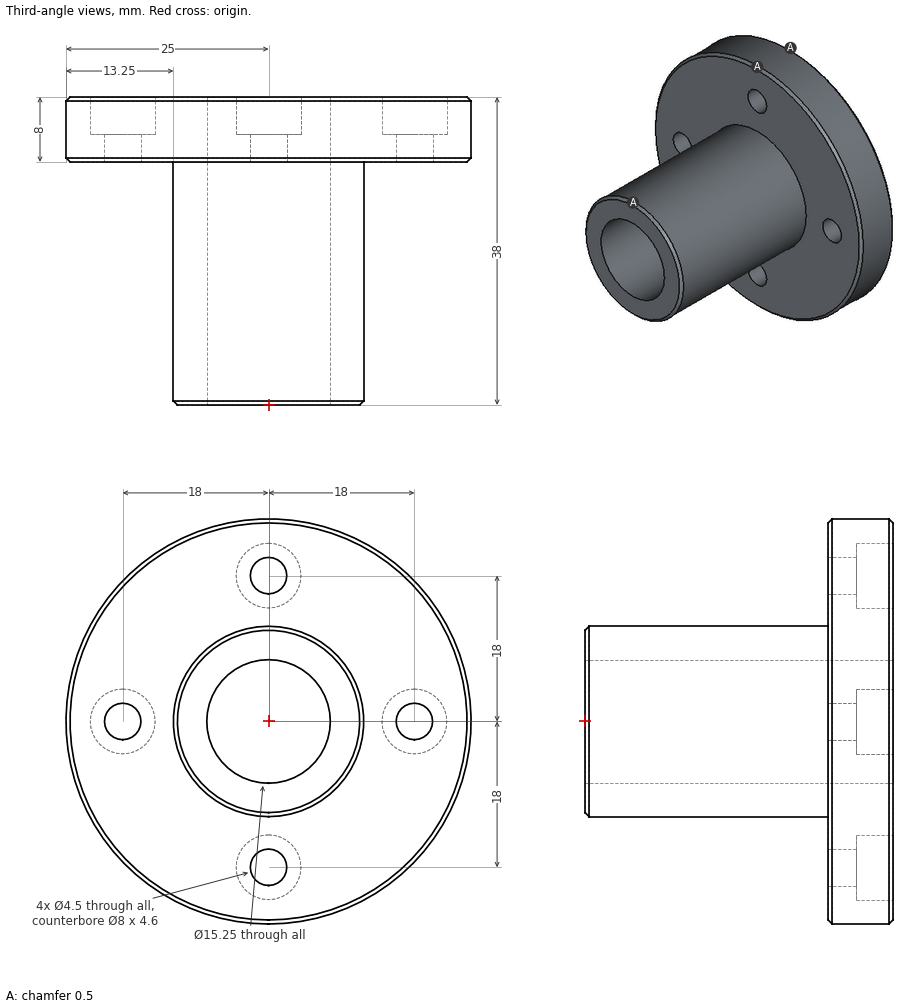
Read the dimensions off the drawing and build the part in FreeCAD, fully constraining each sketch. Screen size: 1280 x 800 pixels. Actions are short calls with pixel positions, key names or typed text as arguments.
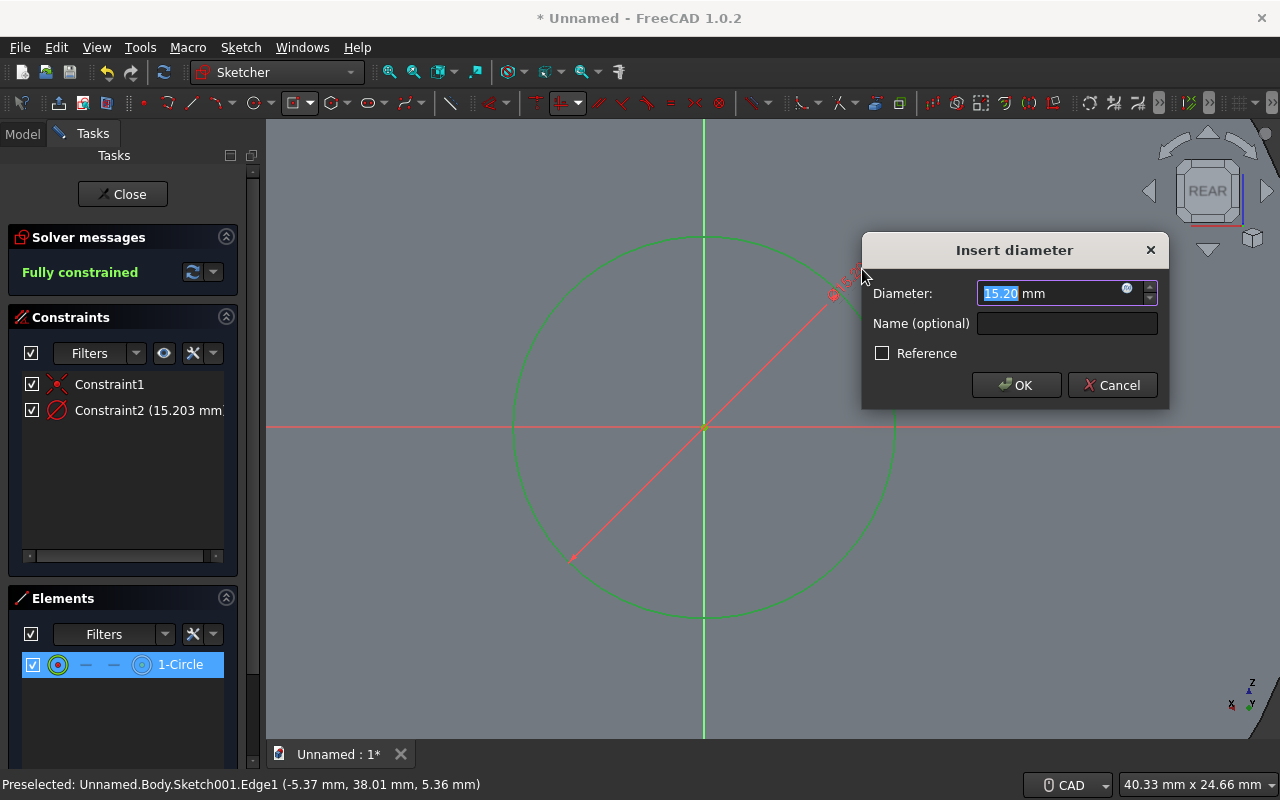
text(15.25)
key(Return)
key(Escape)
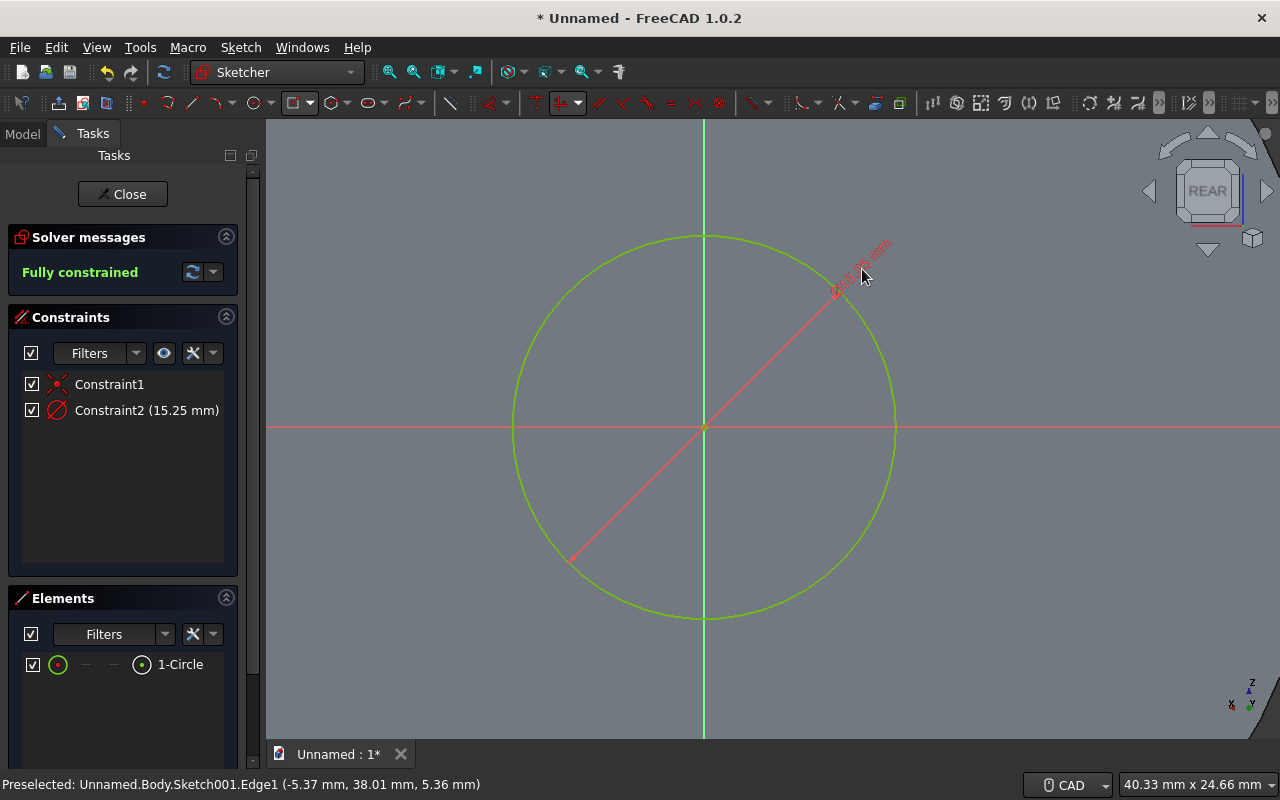
click(123, 194)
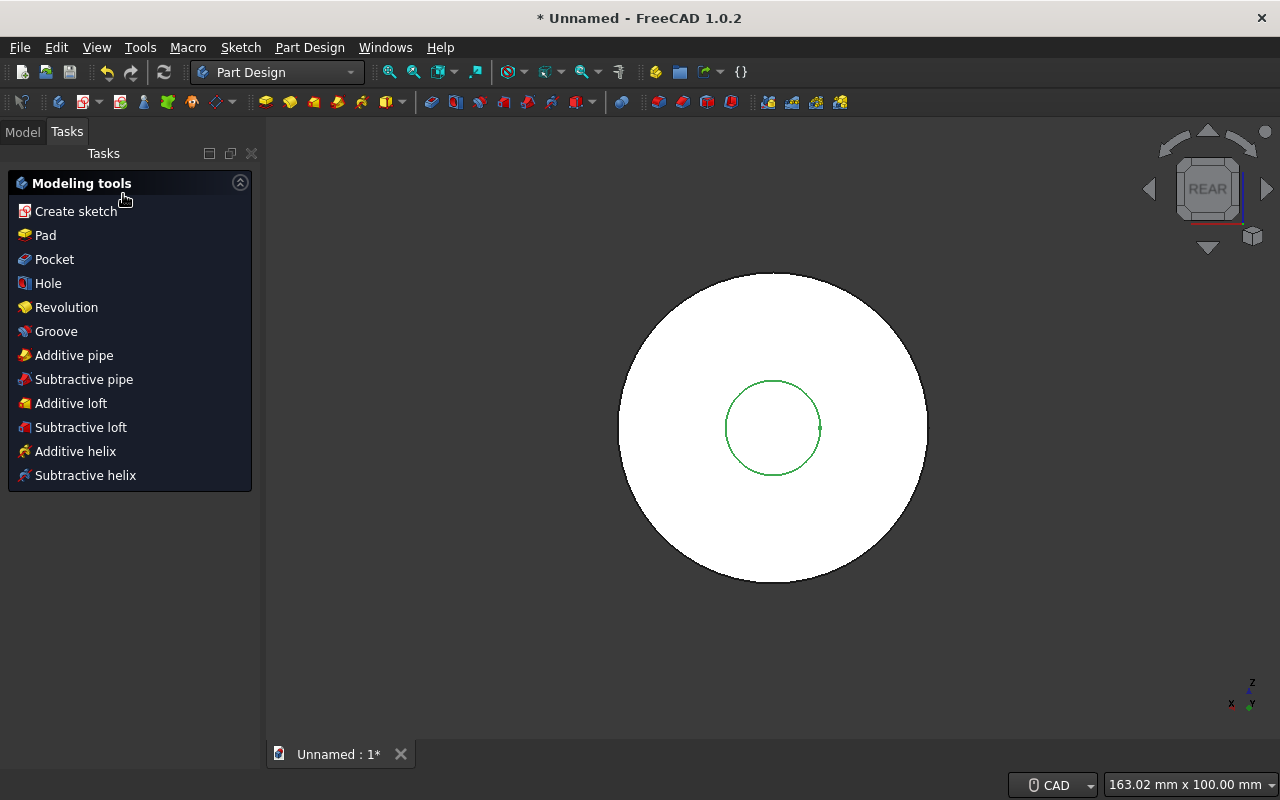
click(456, 102)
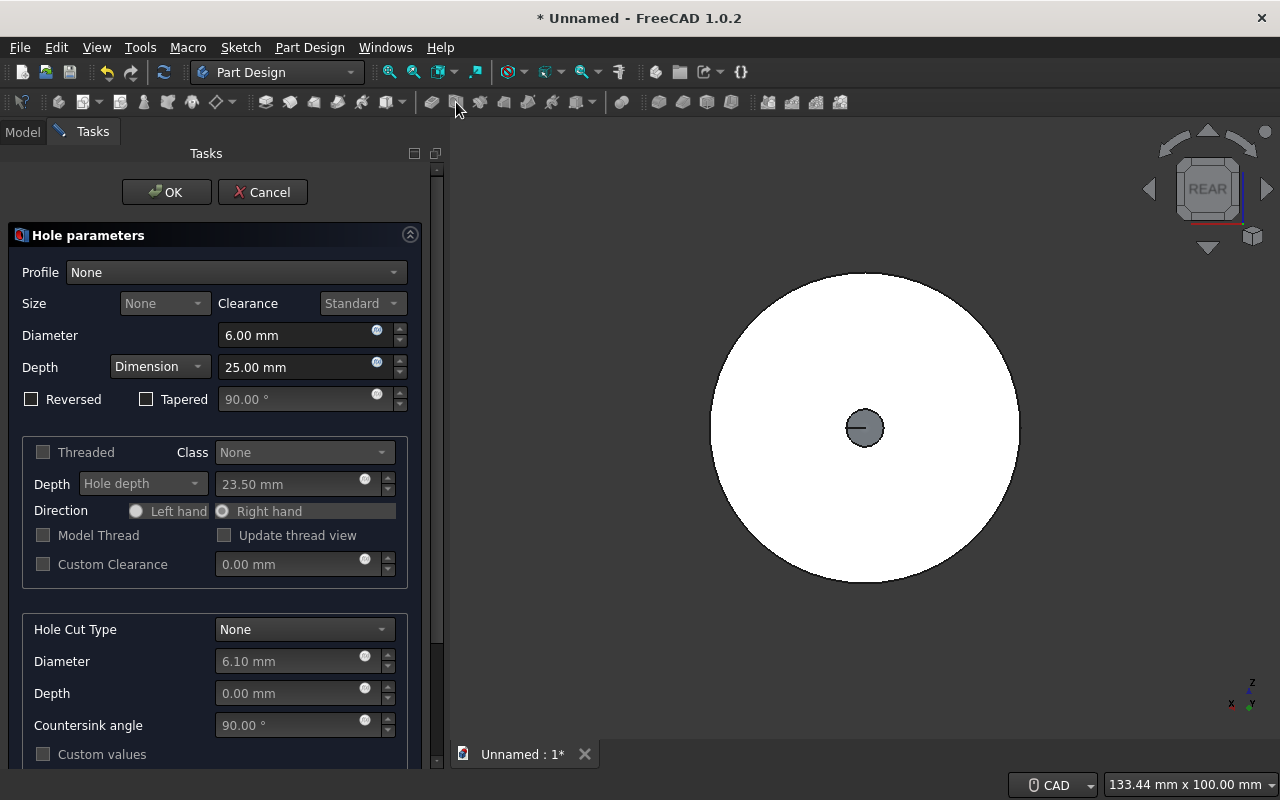
triple_click(305, 335)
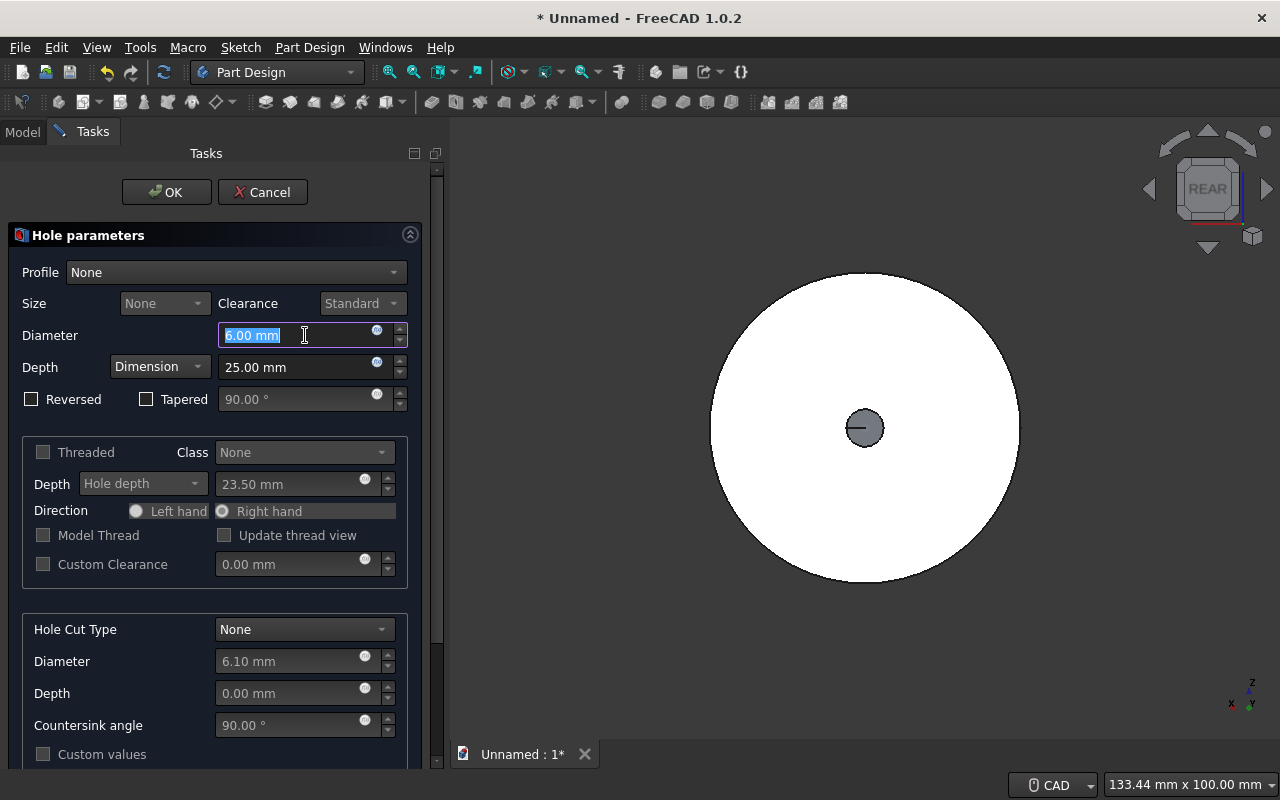
text(15.25)
key(Tab)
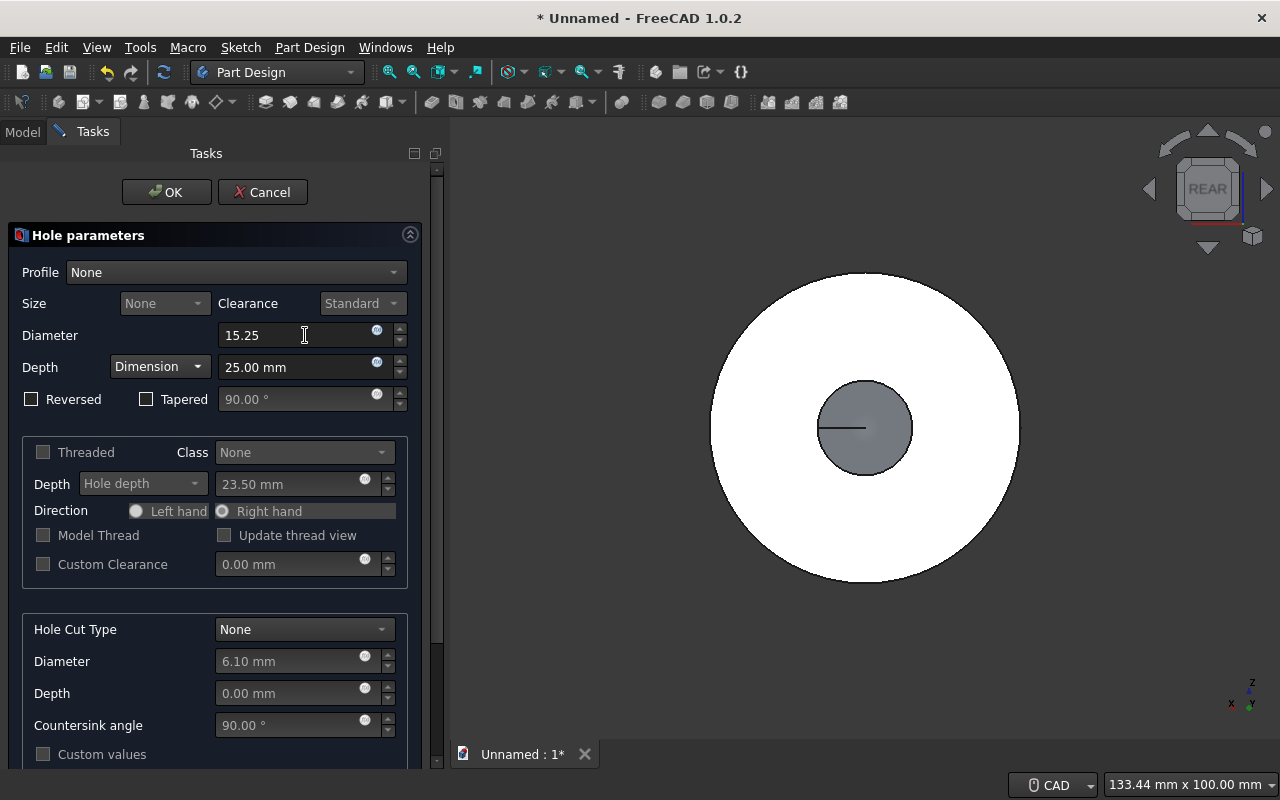
click(161, 366)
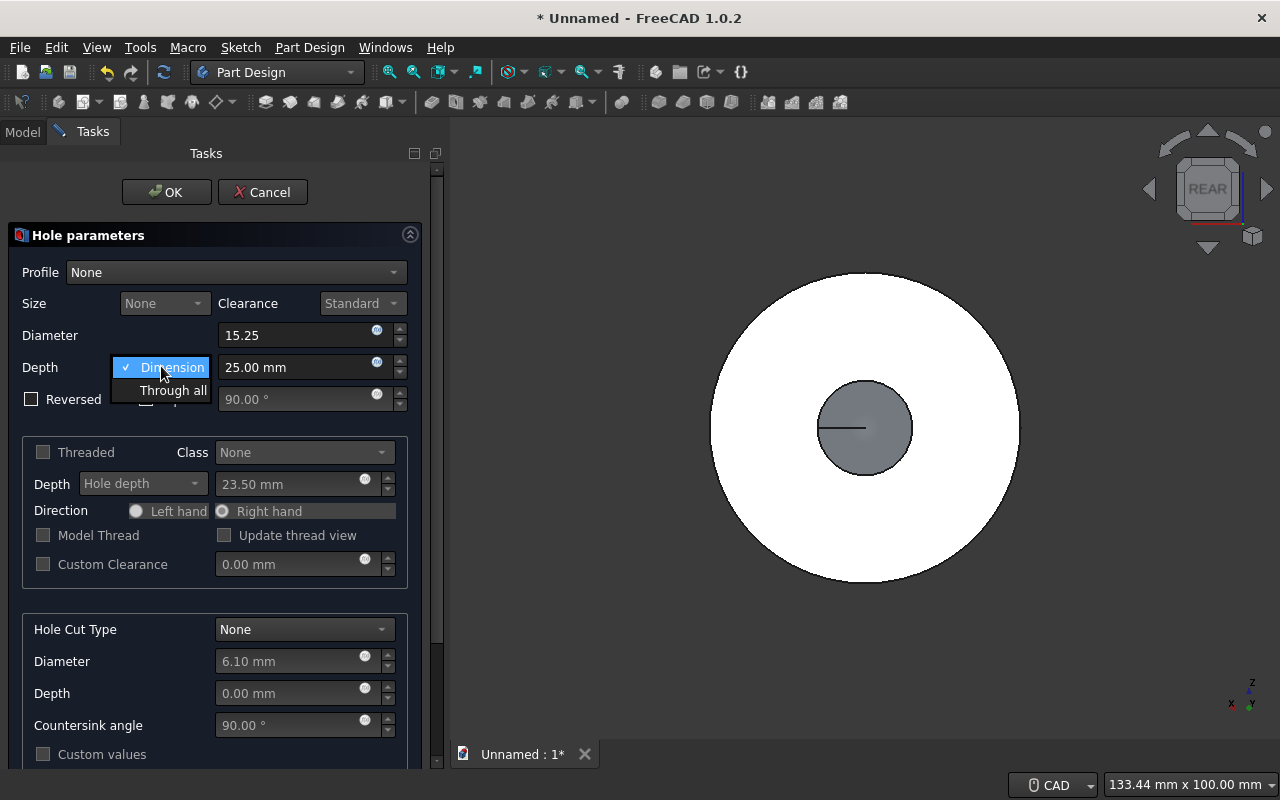
click(160, 390)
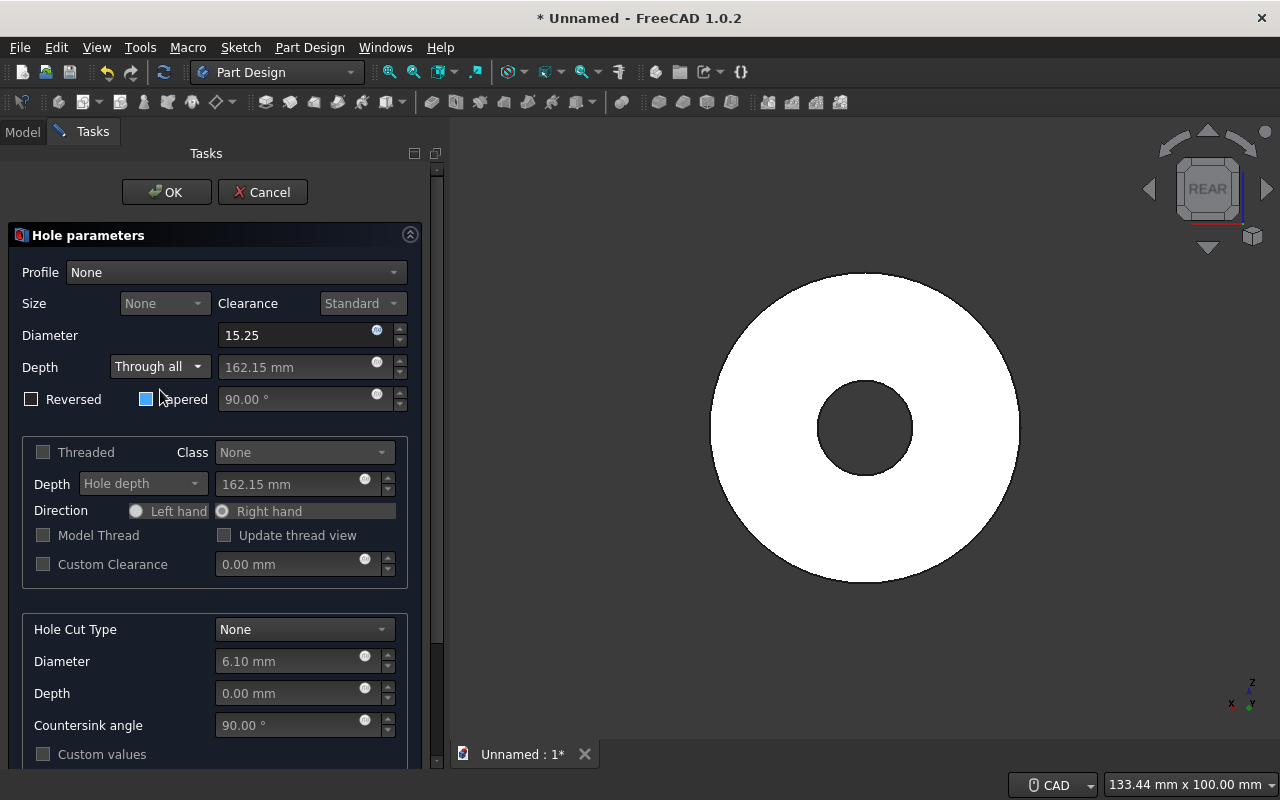
click(167, 192)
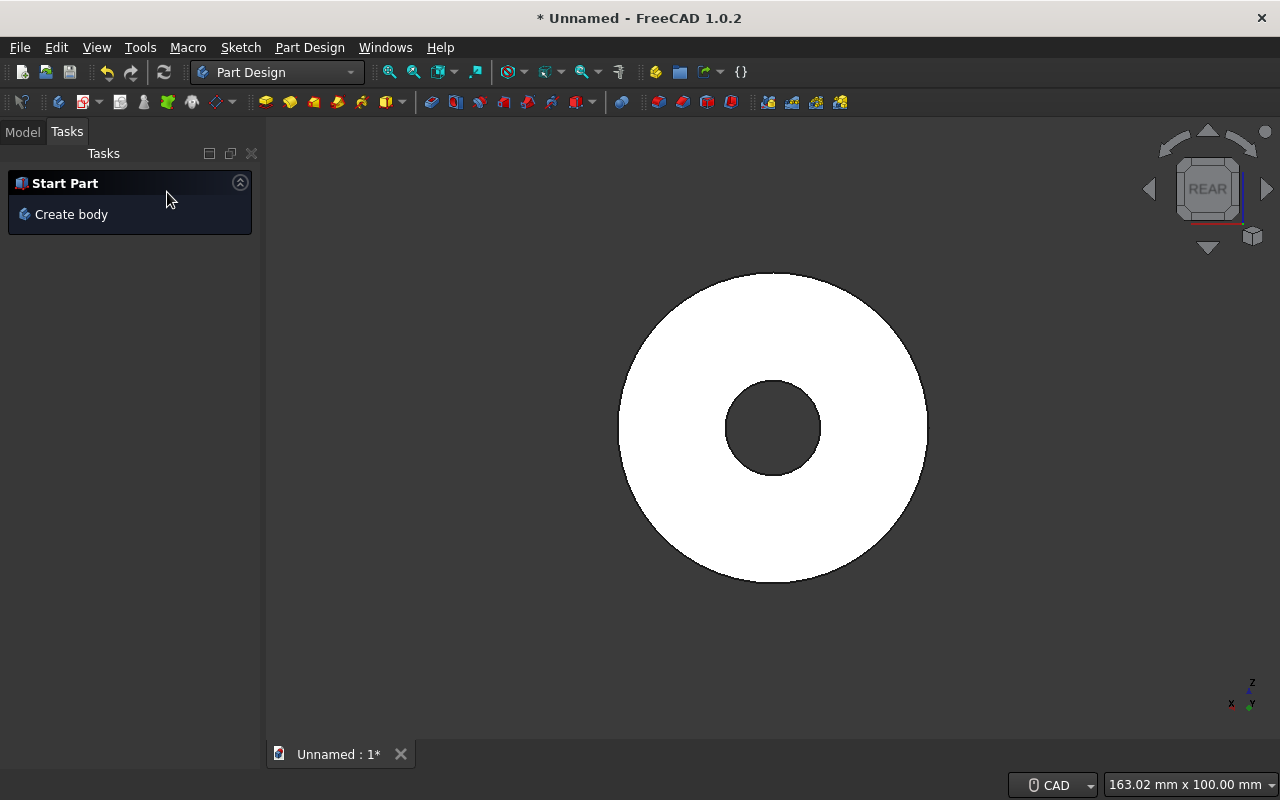
click(684, 383)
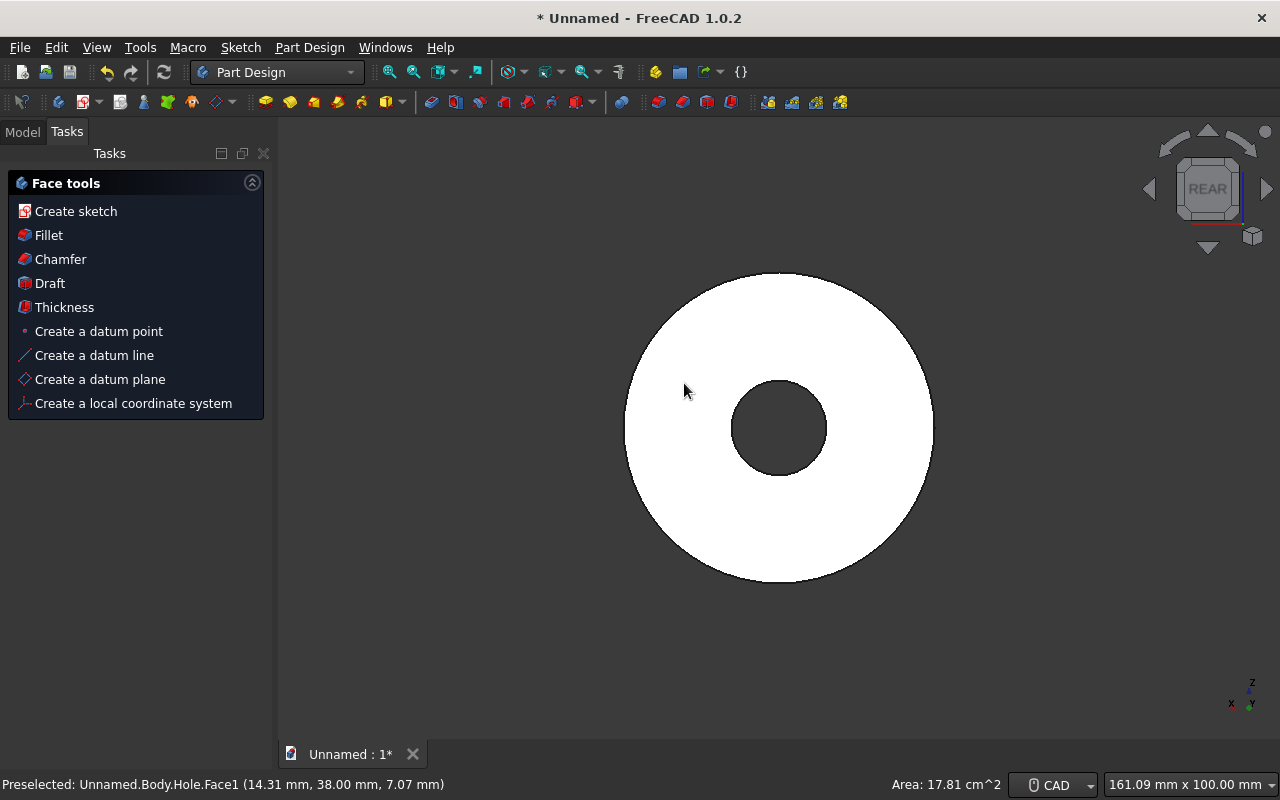
click(84, 102)